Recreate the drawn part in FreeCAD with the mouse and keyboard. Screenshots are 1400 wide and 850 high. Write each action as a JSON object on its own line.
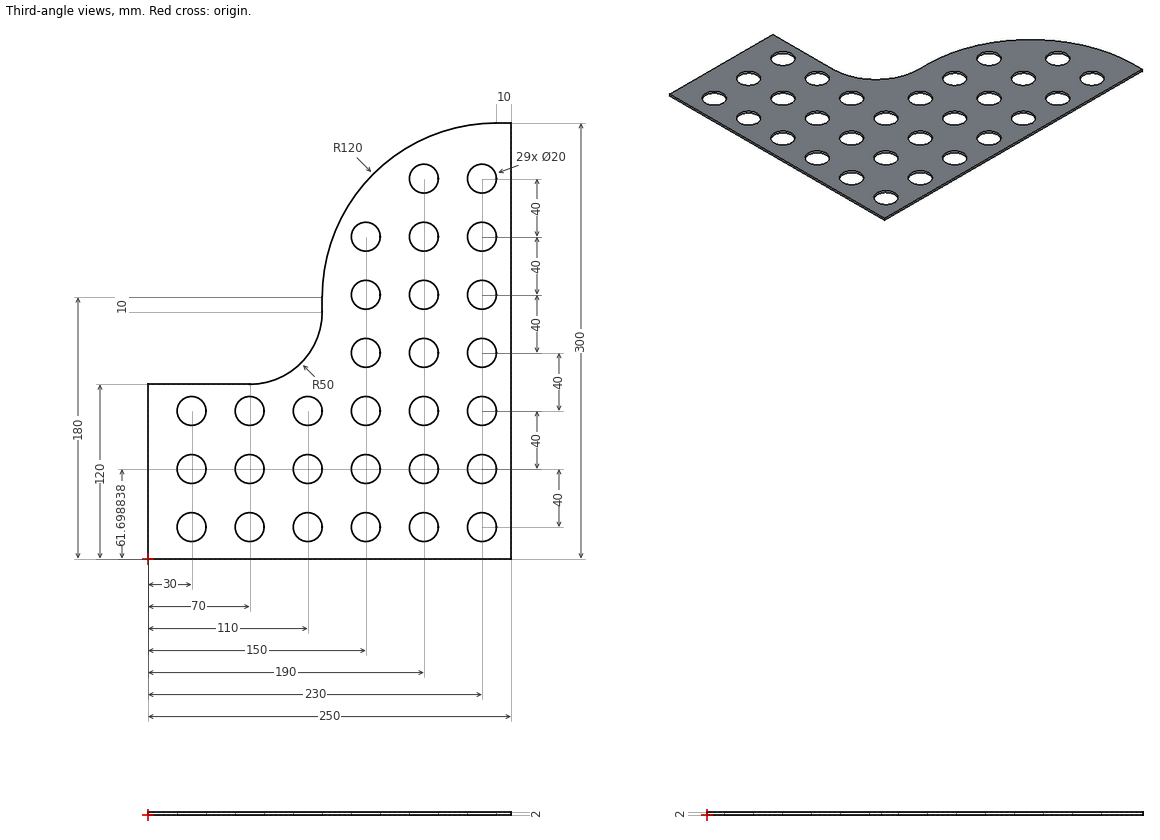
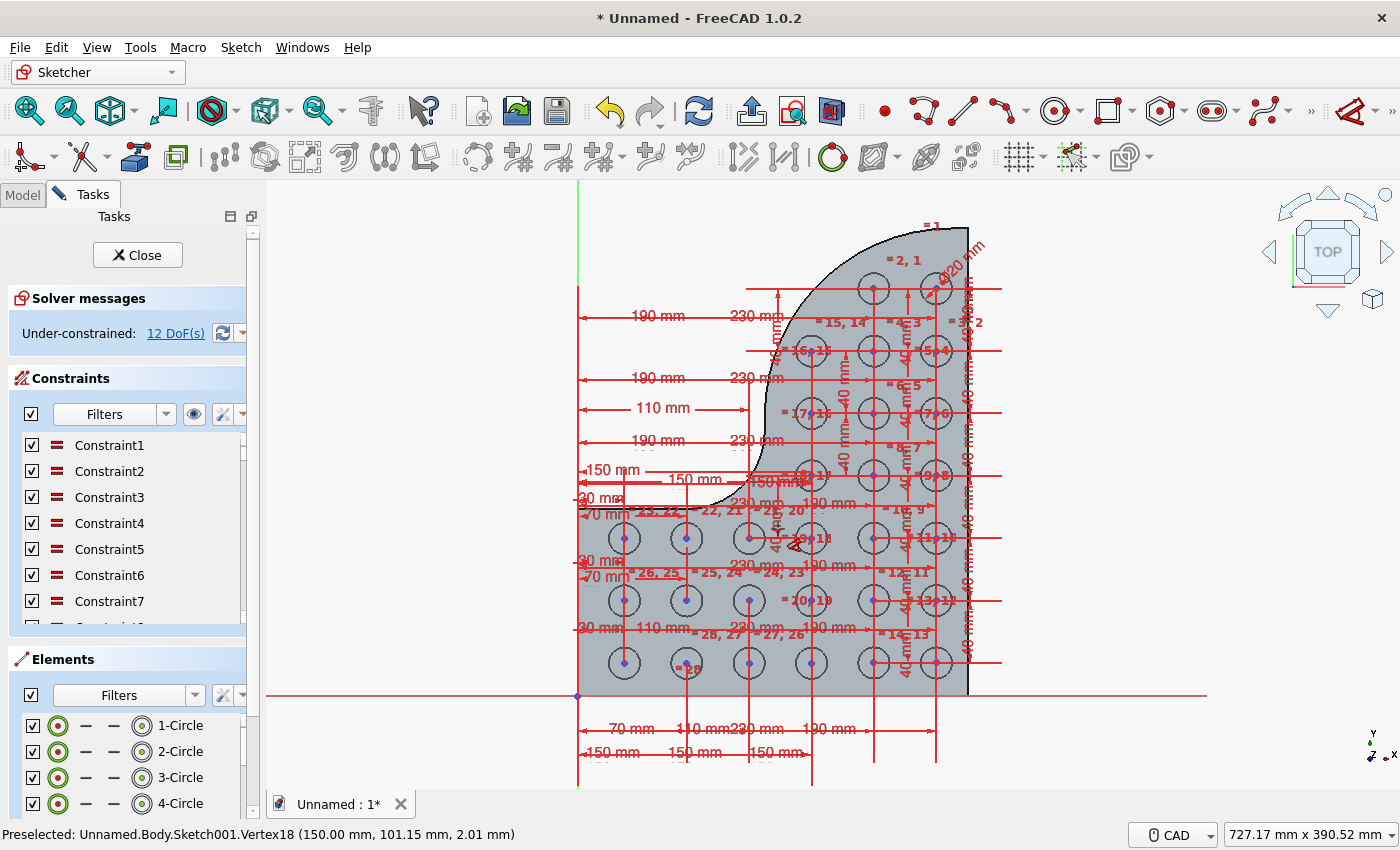
{"action": "left_click", "coordinate": [812, 538]}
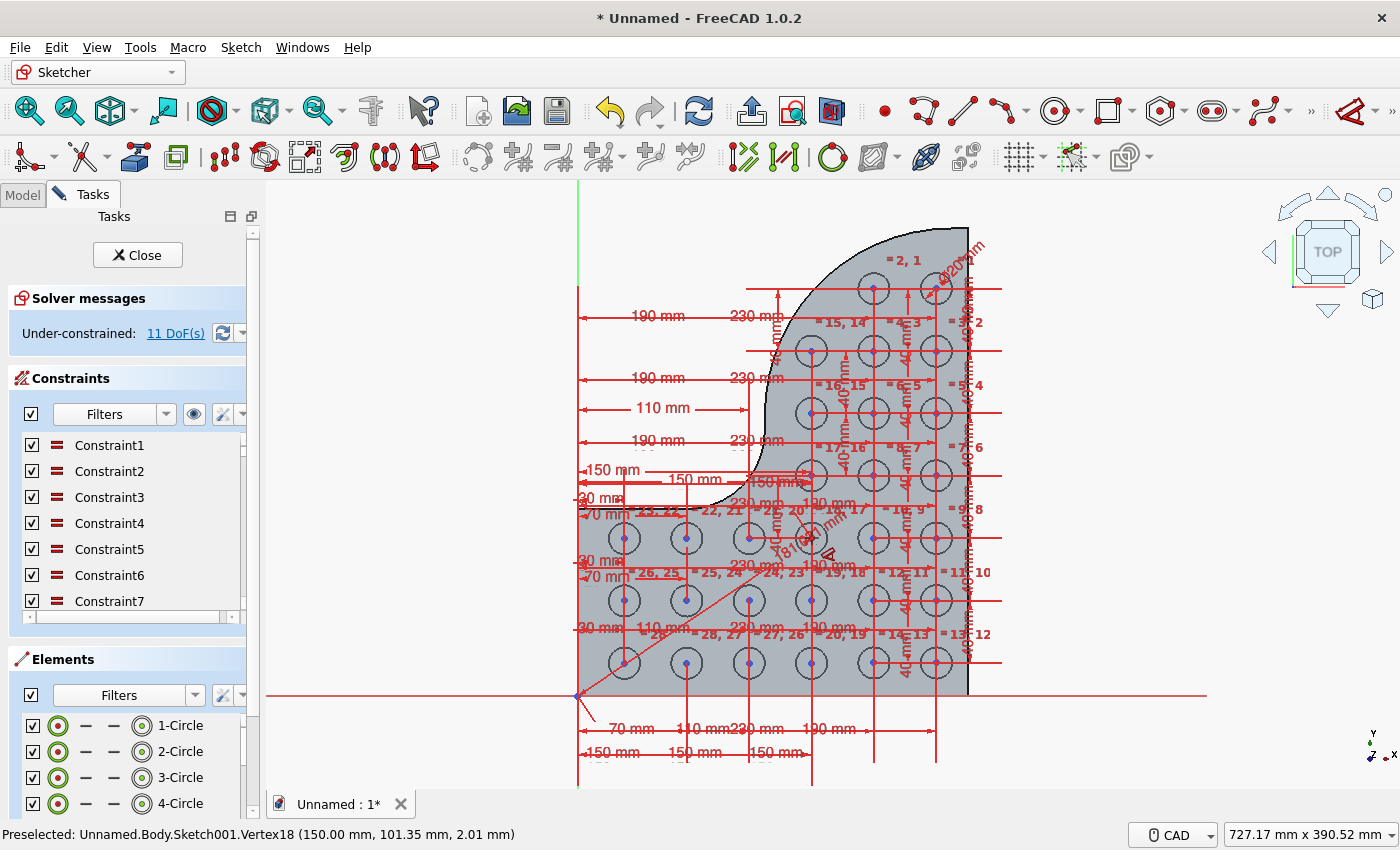
{"action": "left_click", "coordinate": [812, 601]}
{"action": "left_click", "coordinate": [778, 591]}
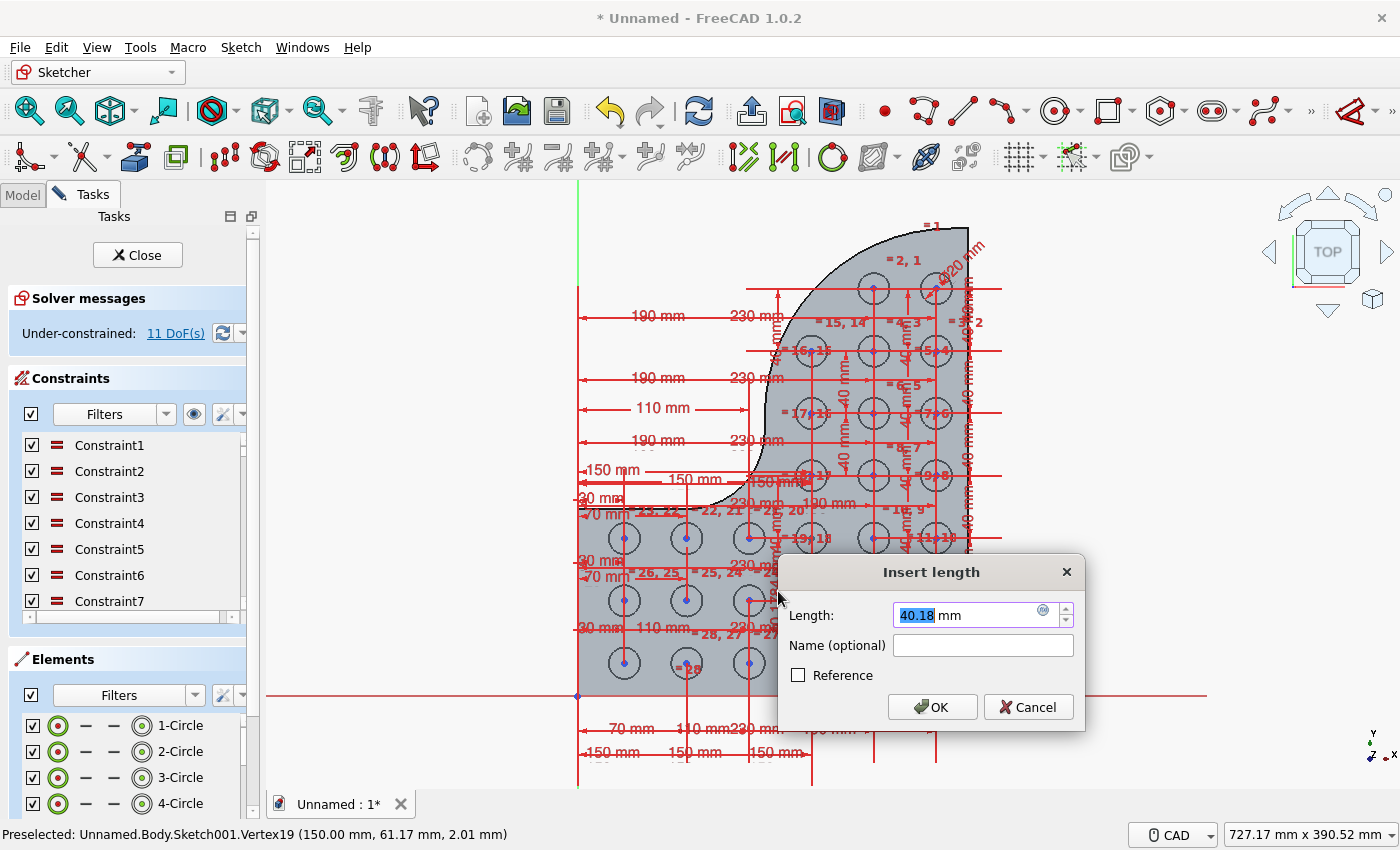
{"action": "type", "text": "40"}
{"action": "key", "text": "Return"}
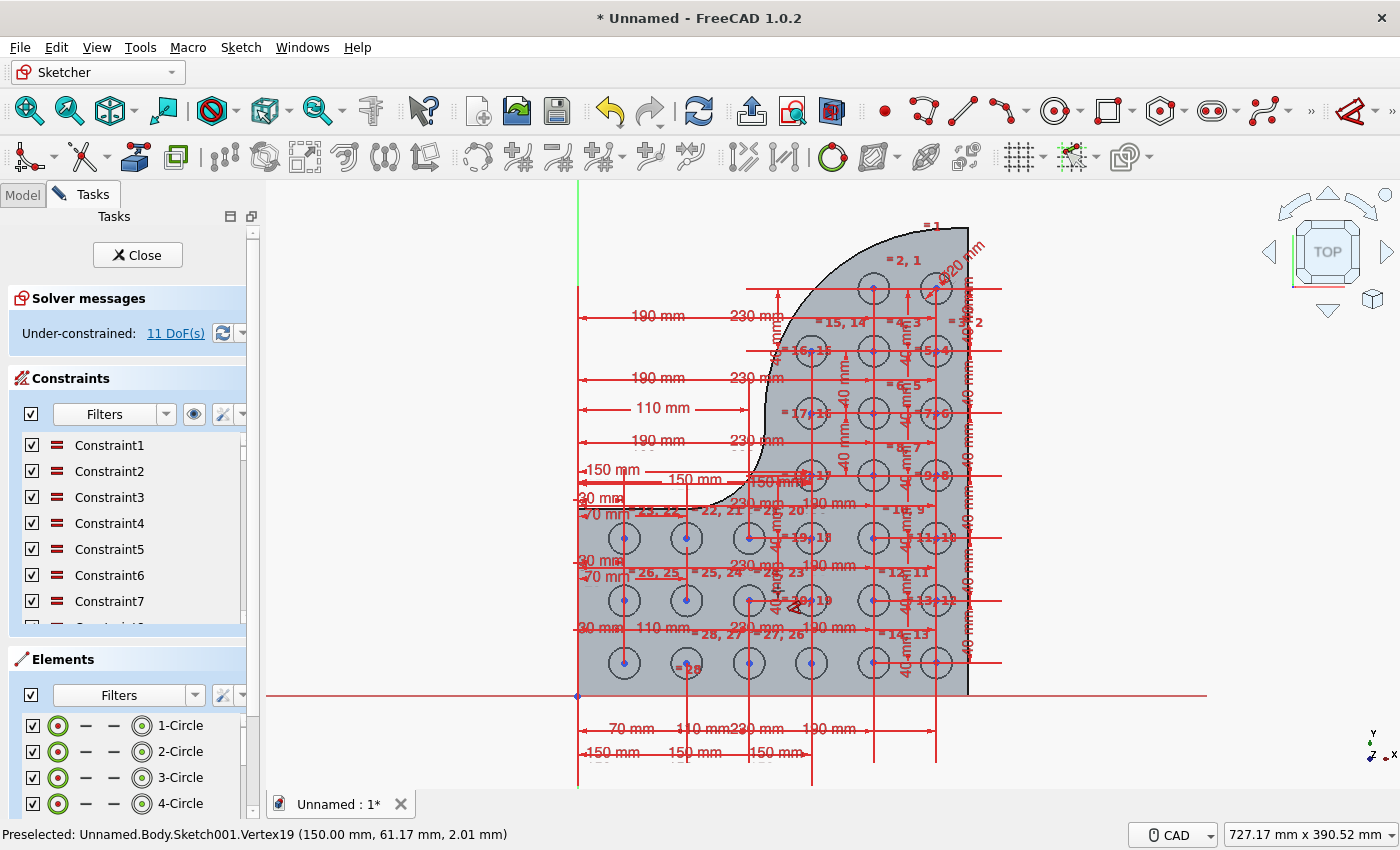
{"action": "left_click", "coordinate": [812, 601]}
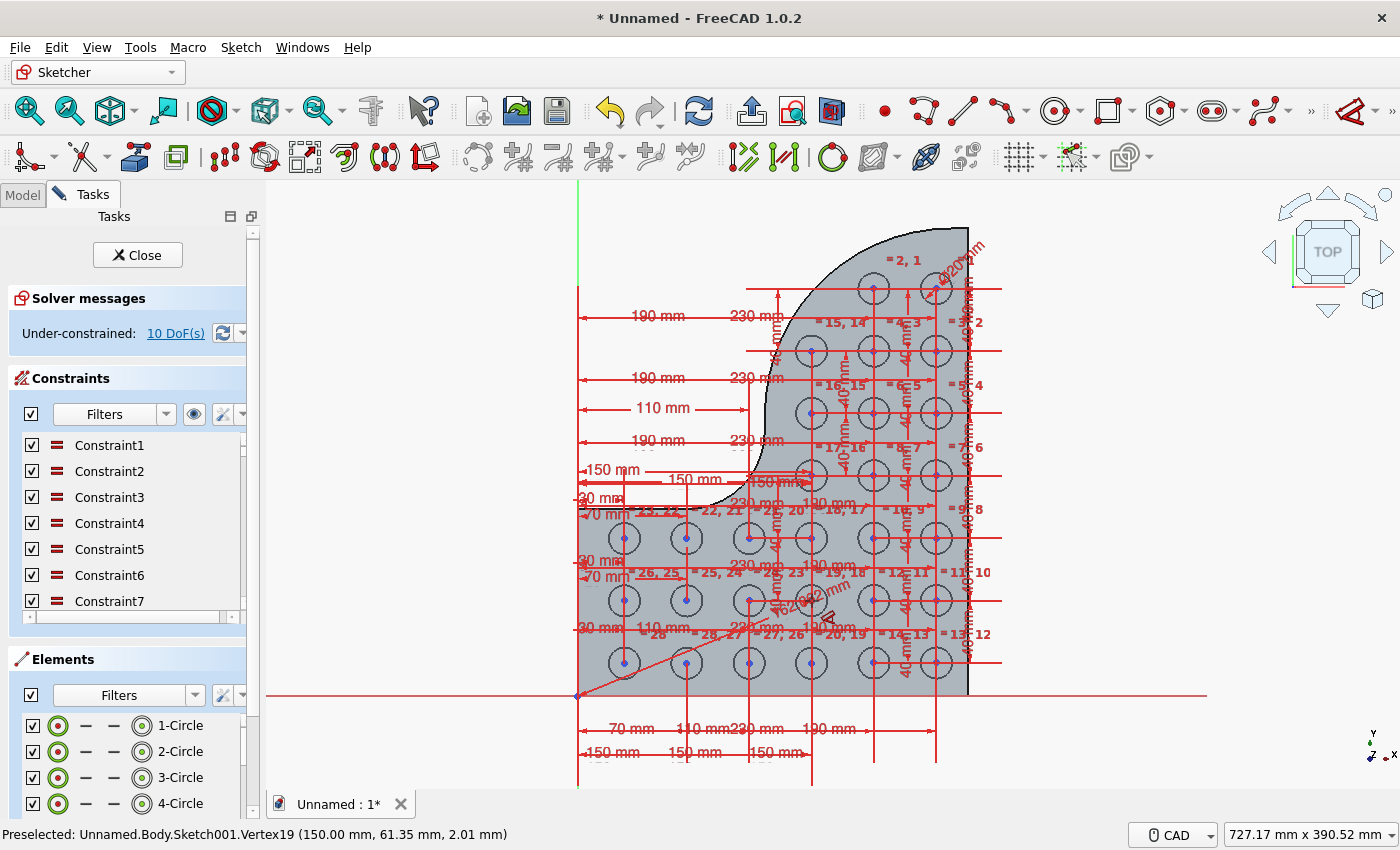
{"action": "left_click", "coordinate": [812, 663]}
{"action": "left_click", "coordinate": [778, 654]}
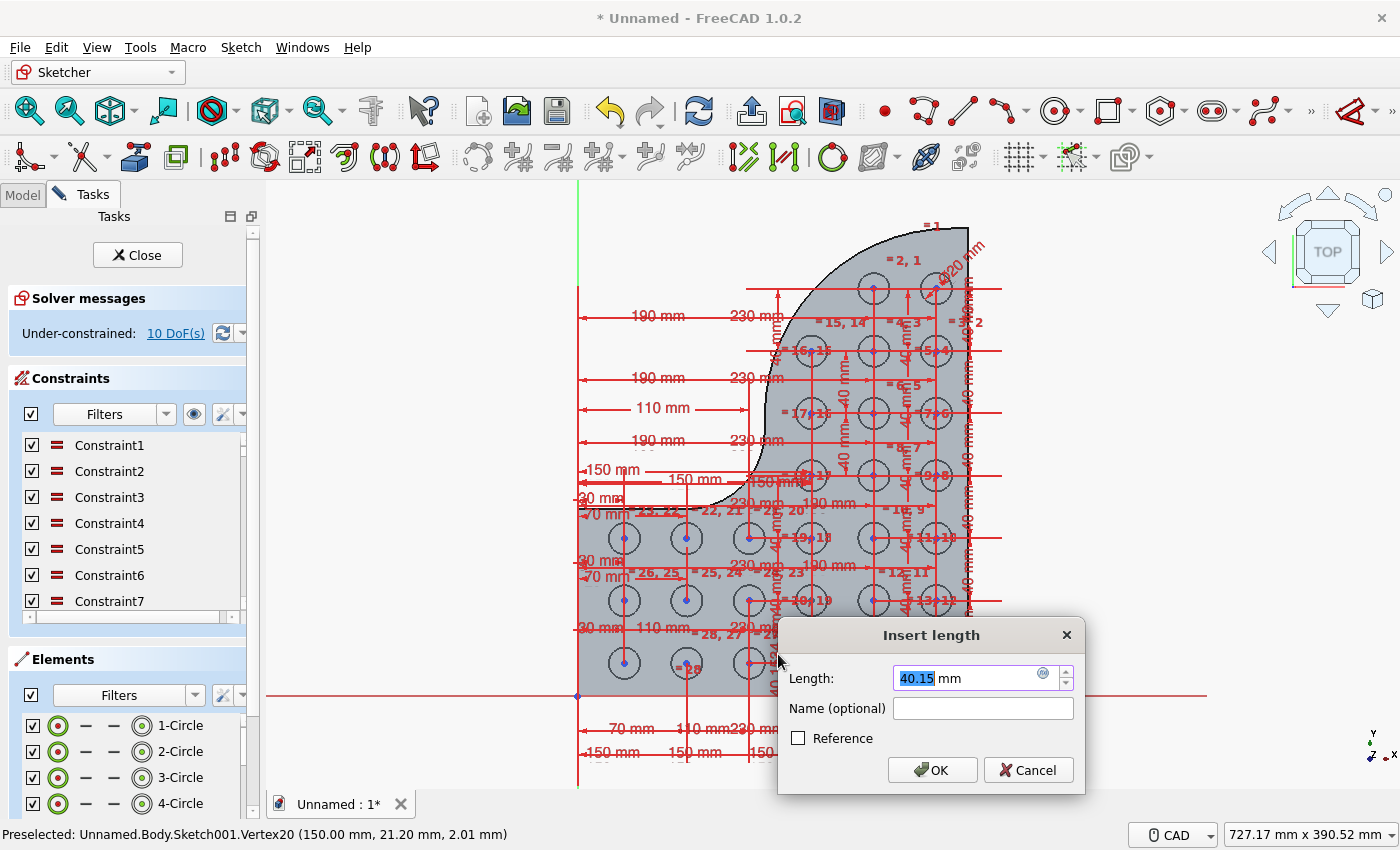
{"action": "type", "text": "40"}
{"action": "key", "text": "Return"}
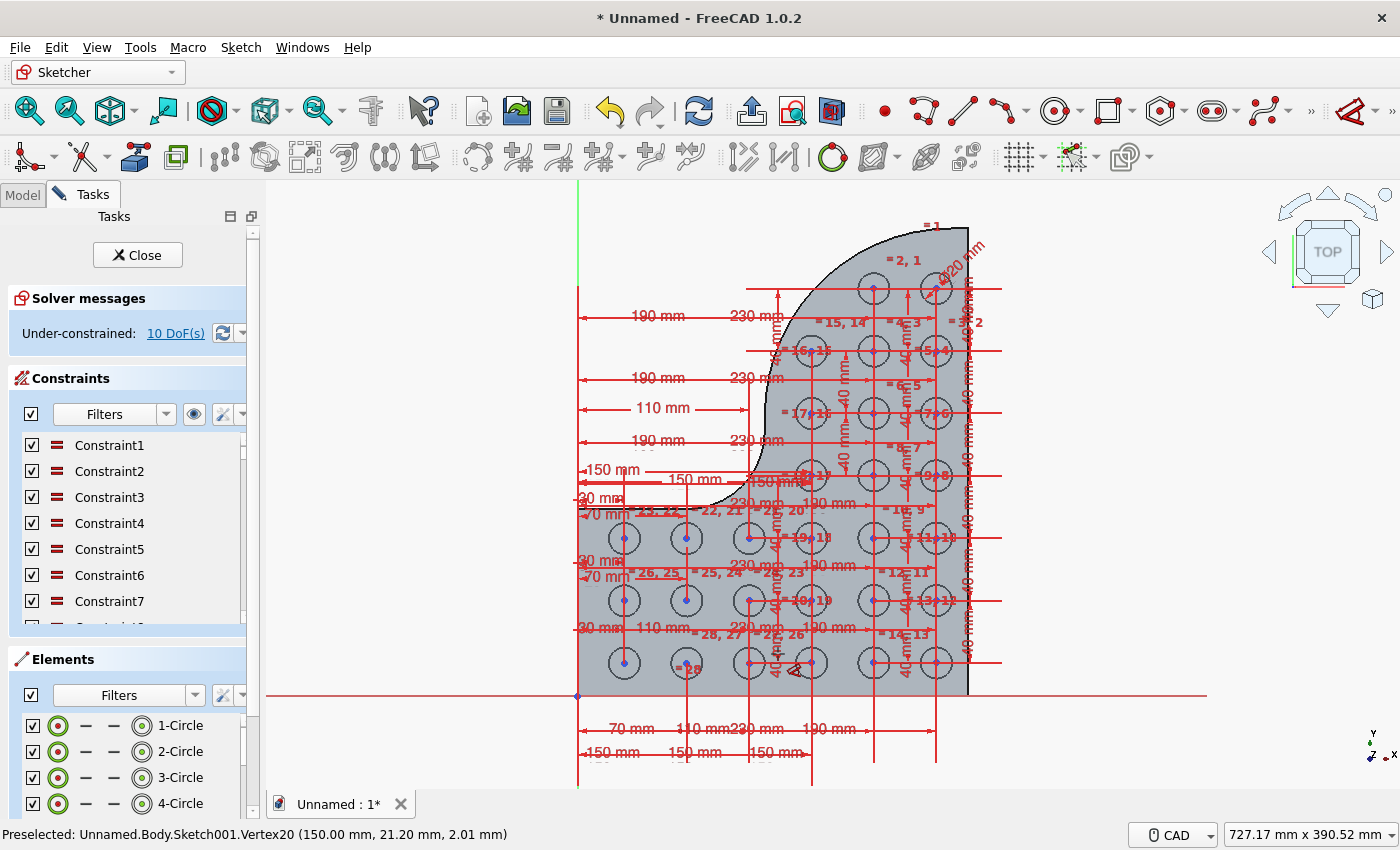
{"action": "left_click", "coordinate": [812, 601]}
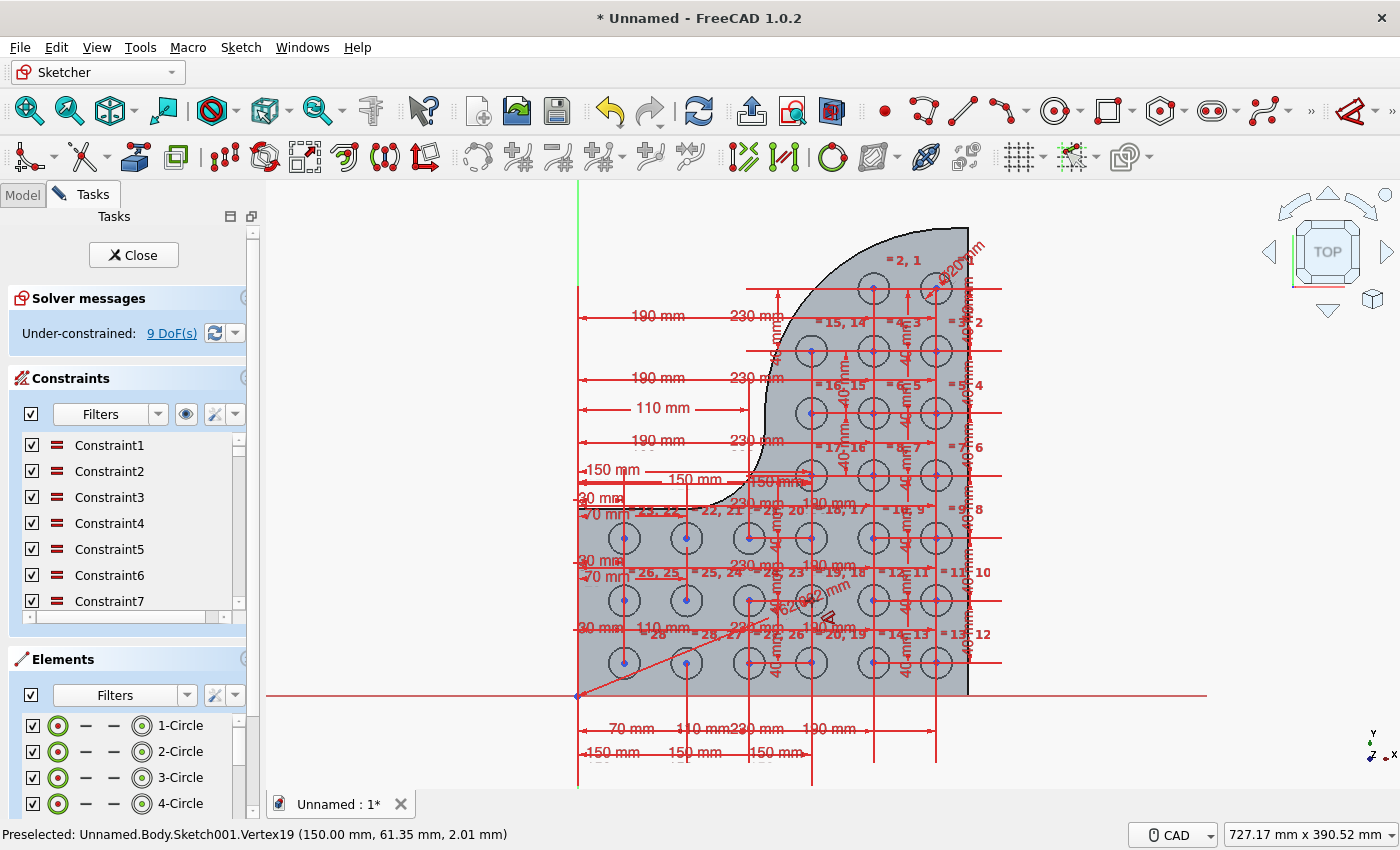
{"action": "left_click", "coordinate": [749, 539]}
{"action": "left_click", "coordinate": [992, 548]}